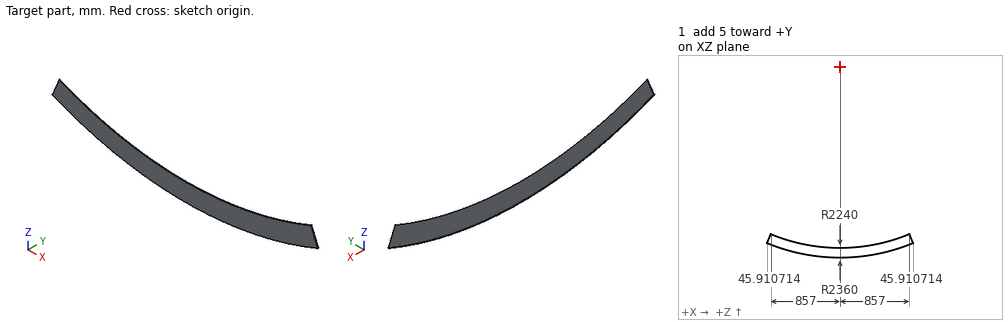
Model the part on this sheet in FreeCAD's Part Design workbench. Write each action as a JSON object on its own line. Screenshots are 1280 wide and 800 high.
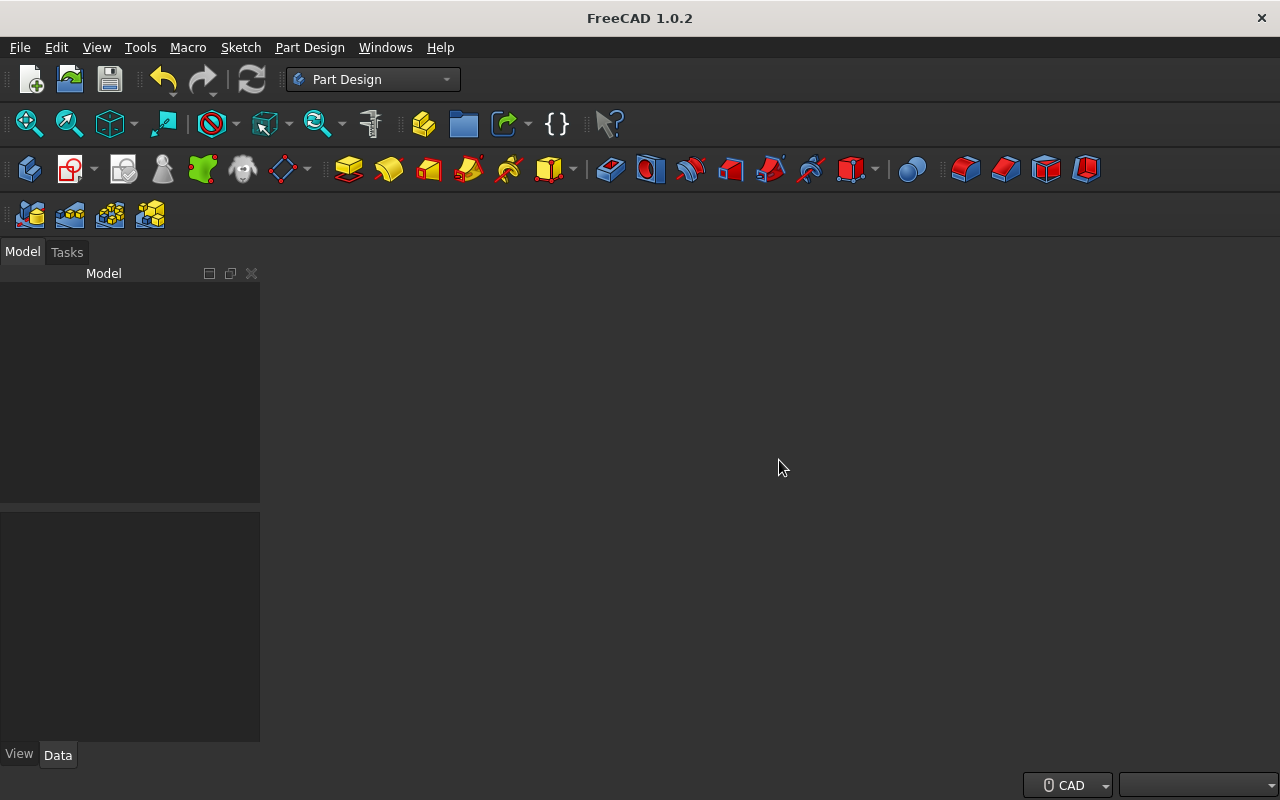
{"action": "left_click", "coordinate": [30, 80]}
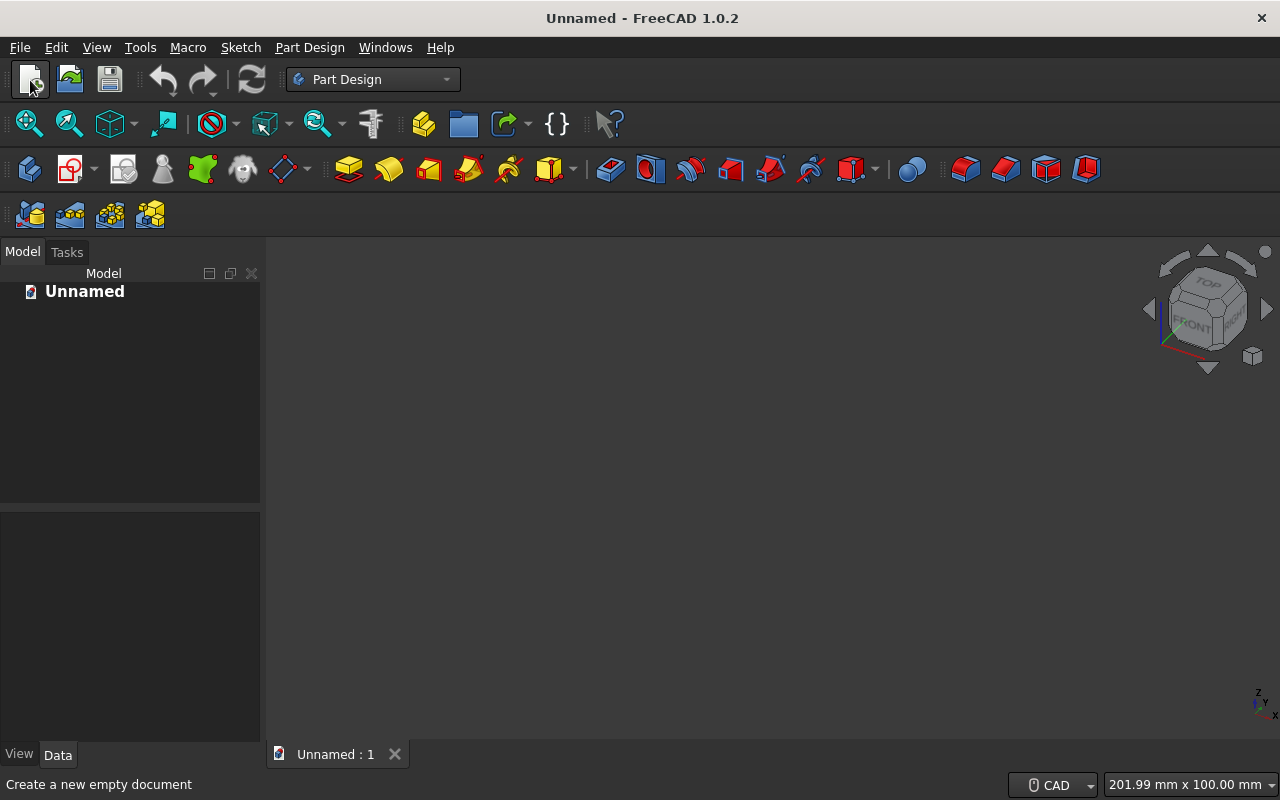
{"action": "left_click", "coordinate": [70, 170]}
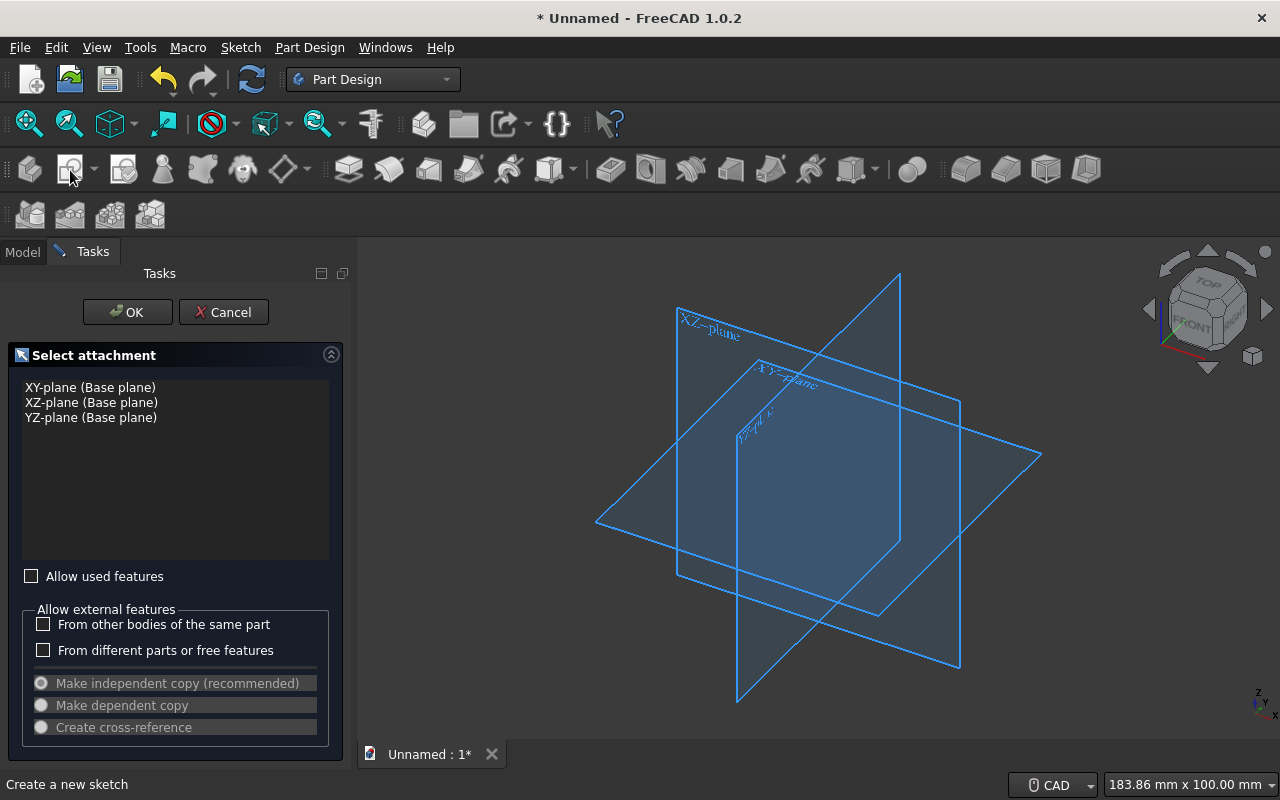
{"action": "left_click", "coordinate": [82, 402]}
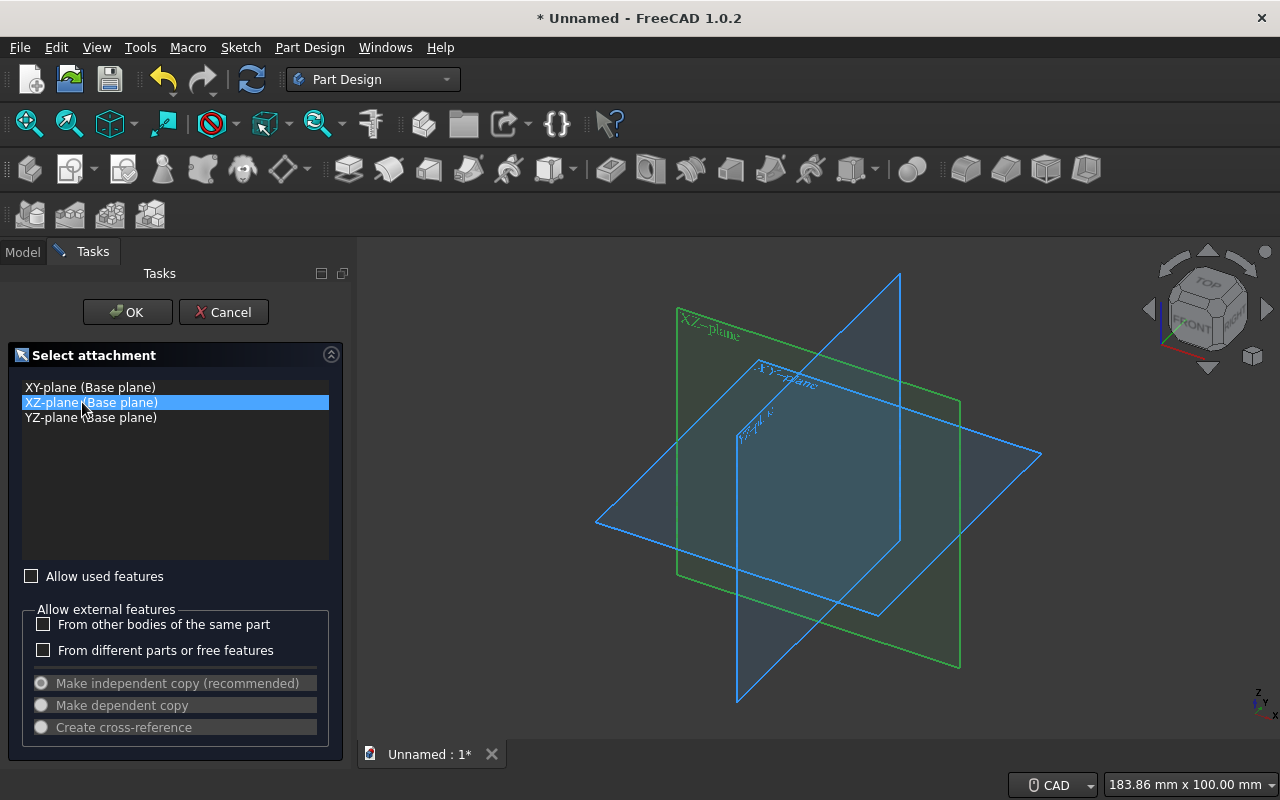
{"action": "left_click", "coordinate": [128, 312]}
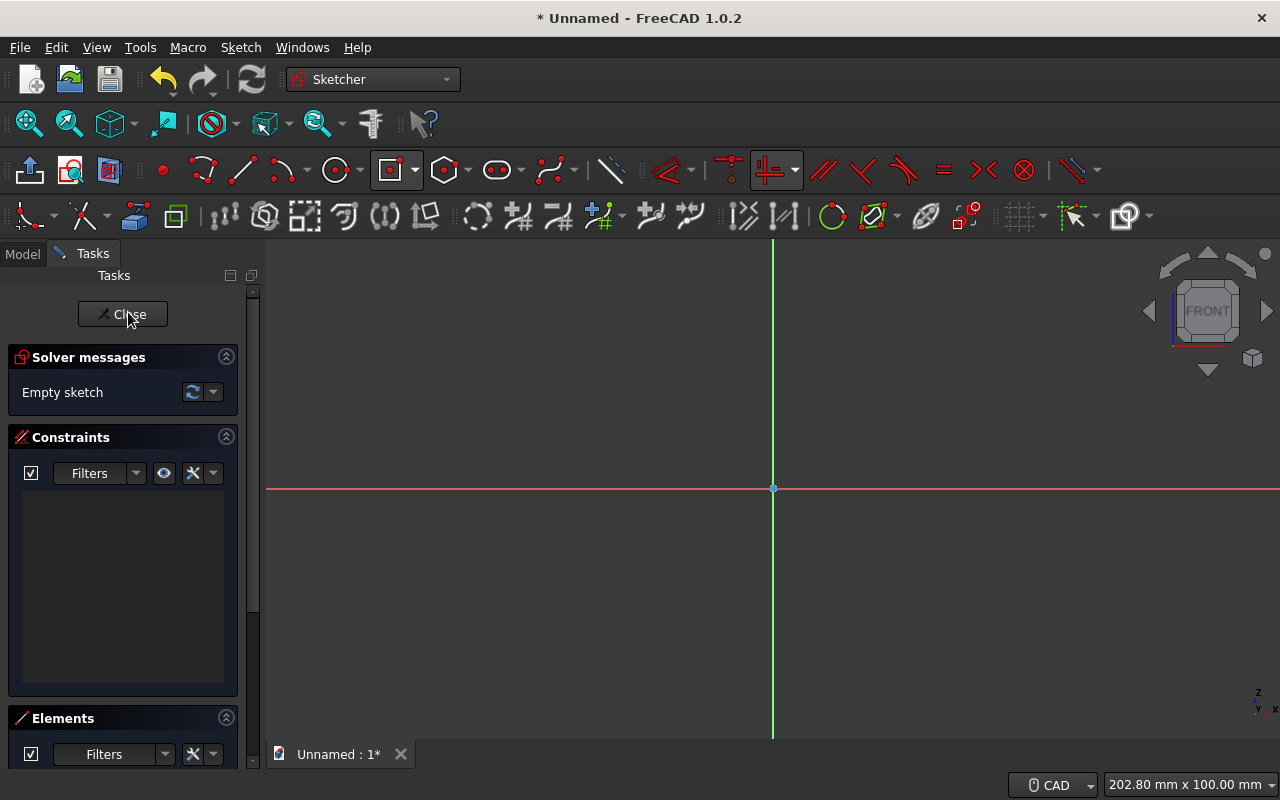
{"action": "scroll", "coordinate": [702, 285], "scroll_direction": "down", "scroll_amount": 17}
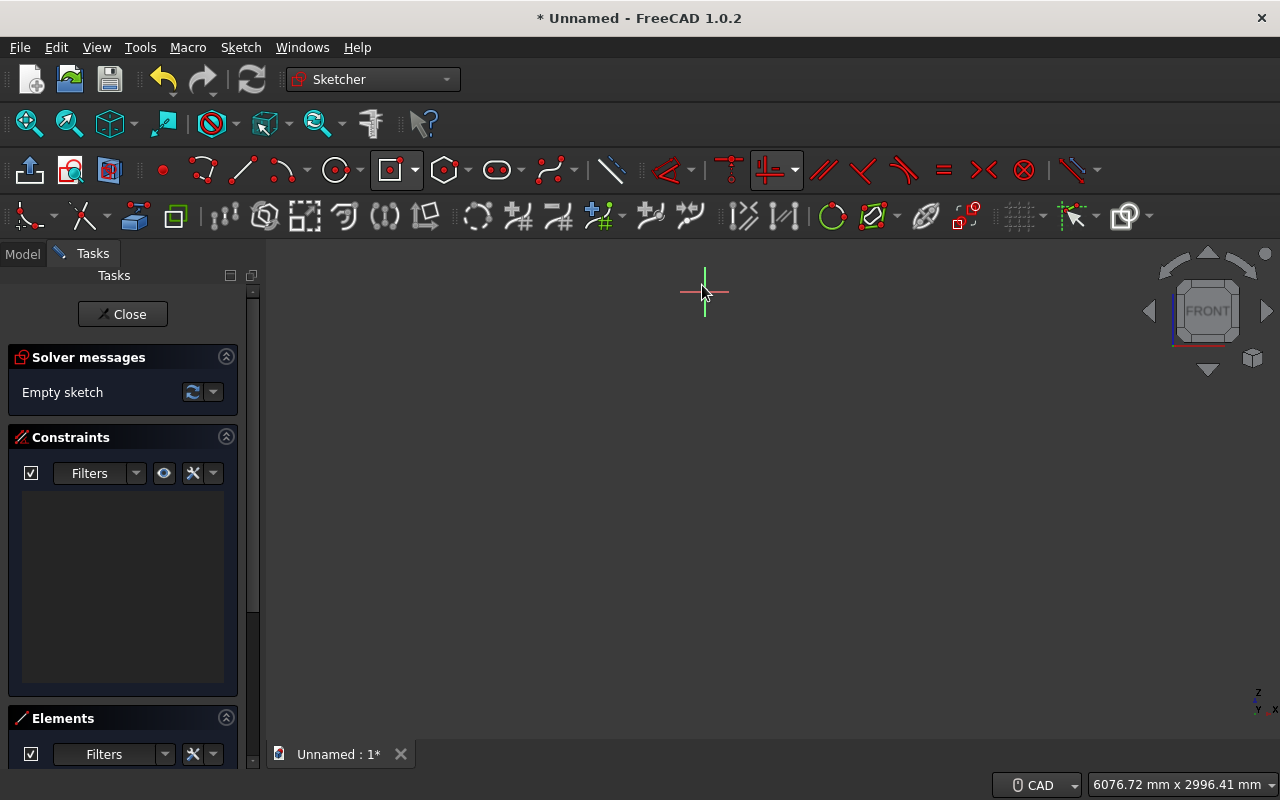
{"action": "scroll", "coordinate": [703, 490], "scroll_direction": "down", "scroll_amount": 1}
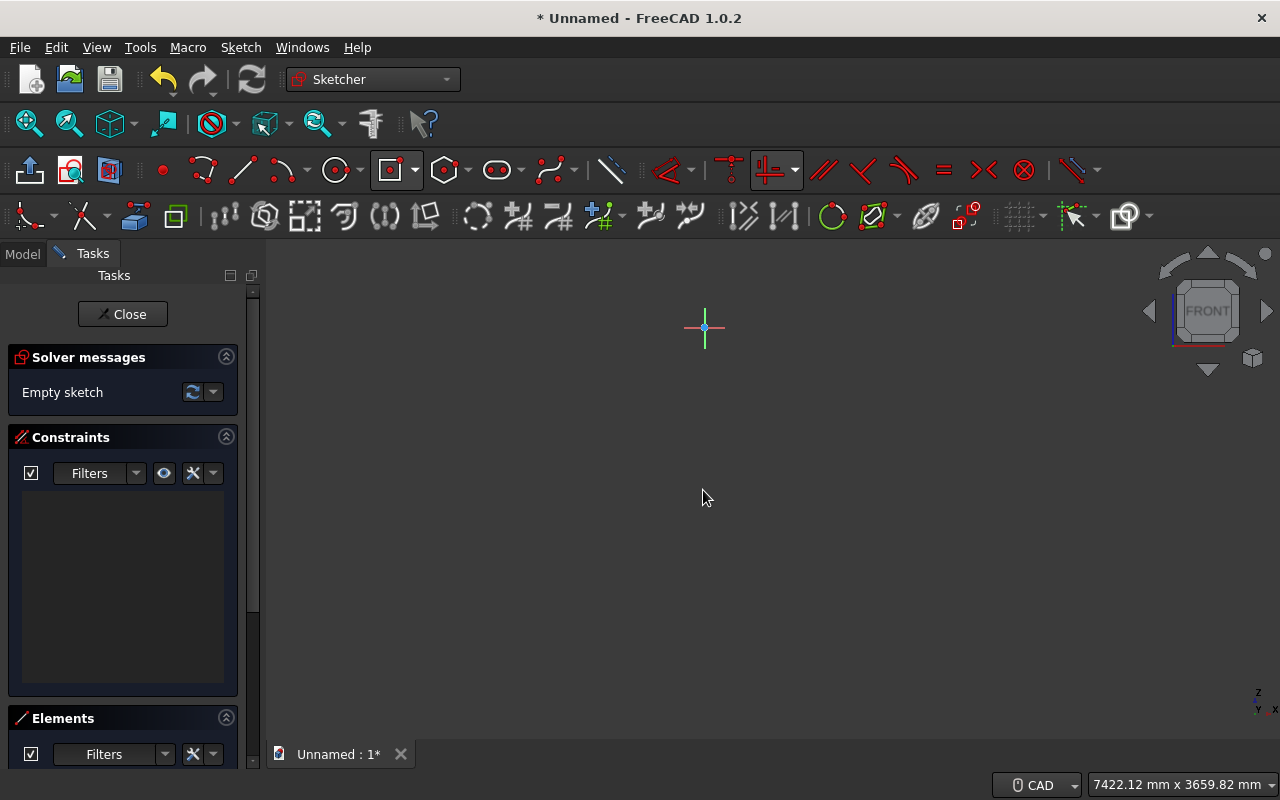
{"action": "left_click", "coordinate": [244, 170]}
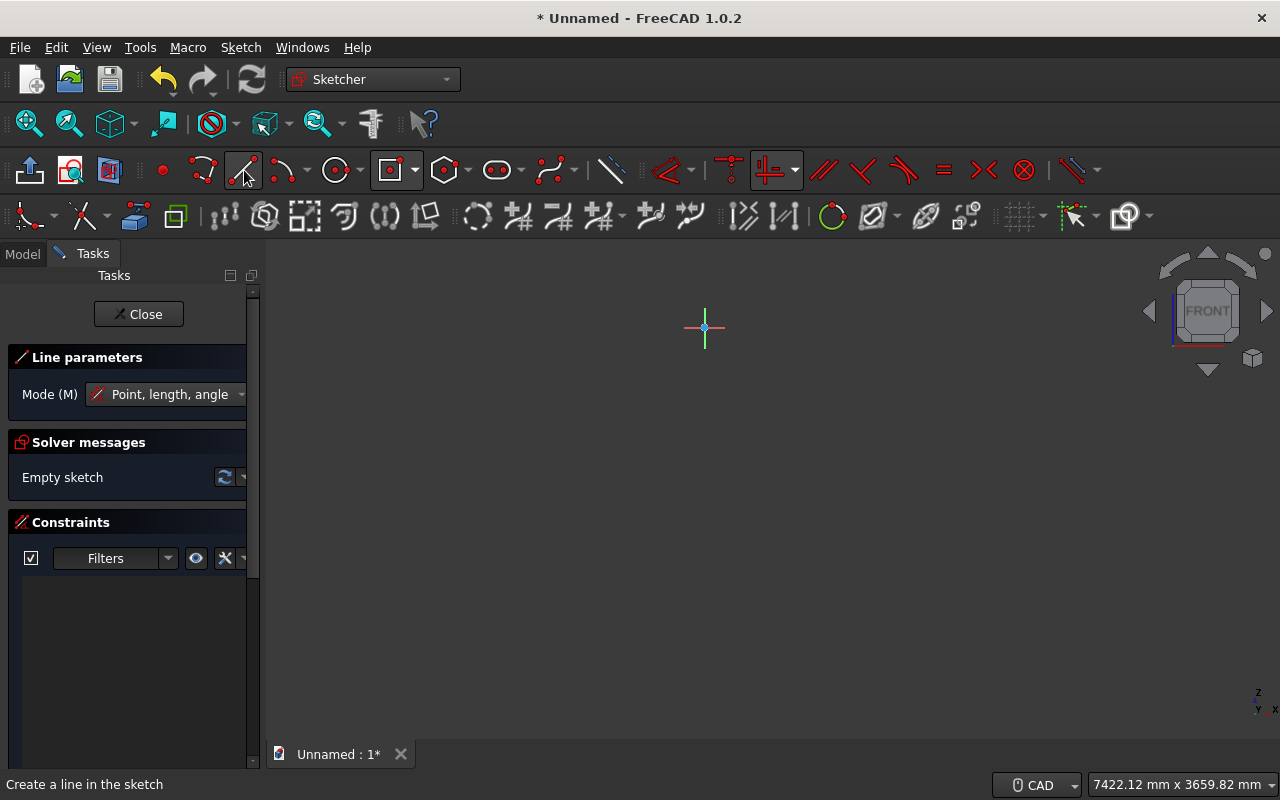
{"action": "left_click", "coordinate": [581, 626]}
{"action": "left_click", "coordinate": [587, 611]}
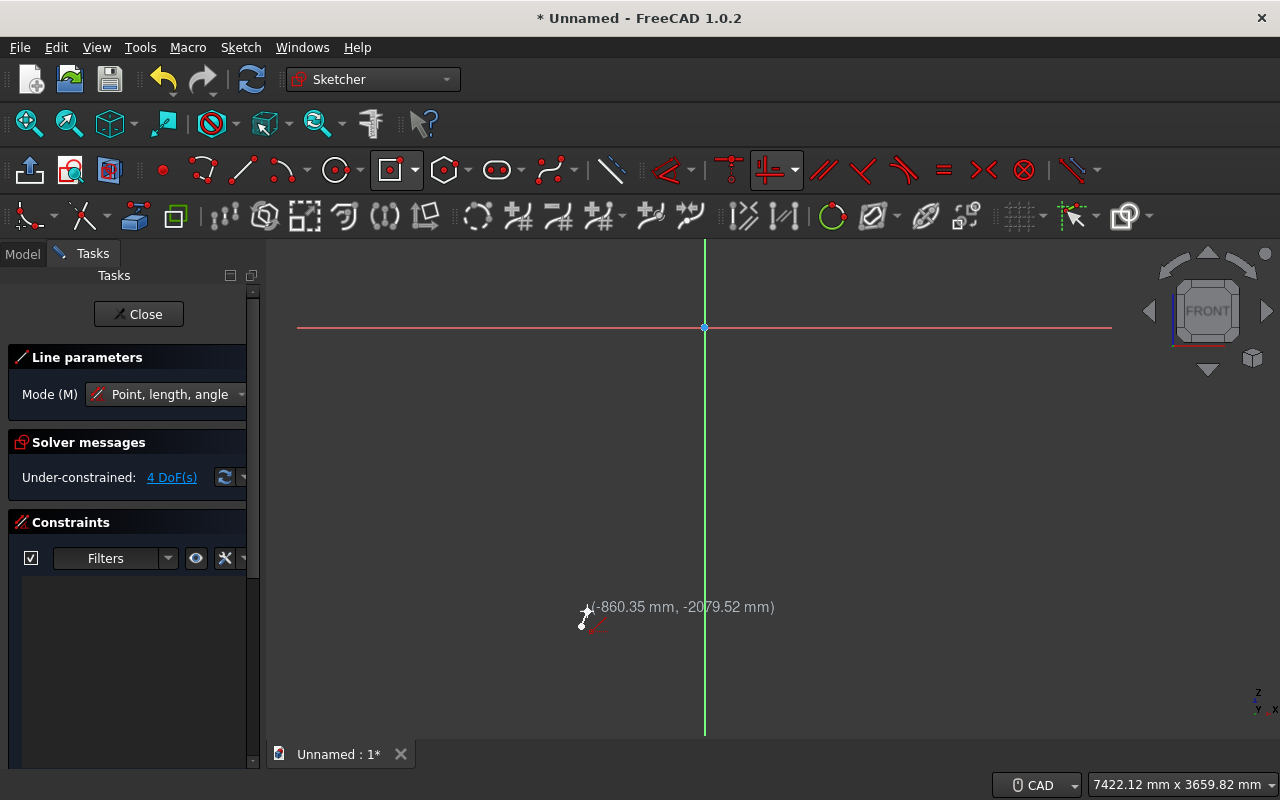
{"action": "left_click", "coordinate": [822, 611]}
{"action": "left_click", "coordinate": [828, 626]}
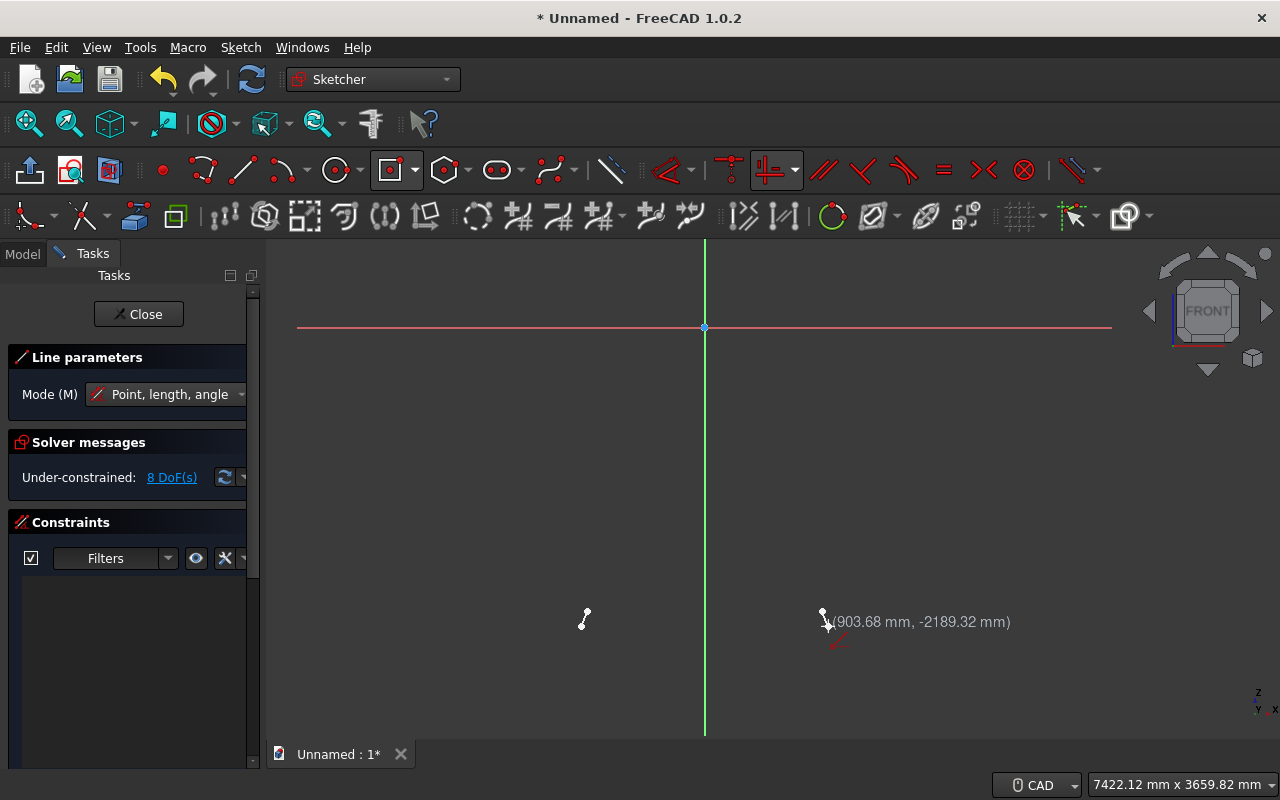
{"action": "left_click", "coordinate": [310, 170]}